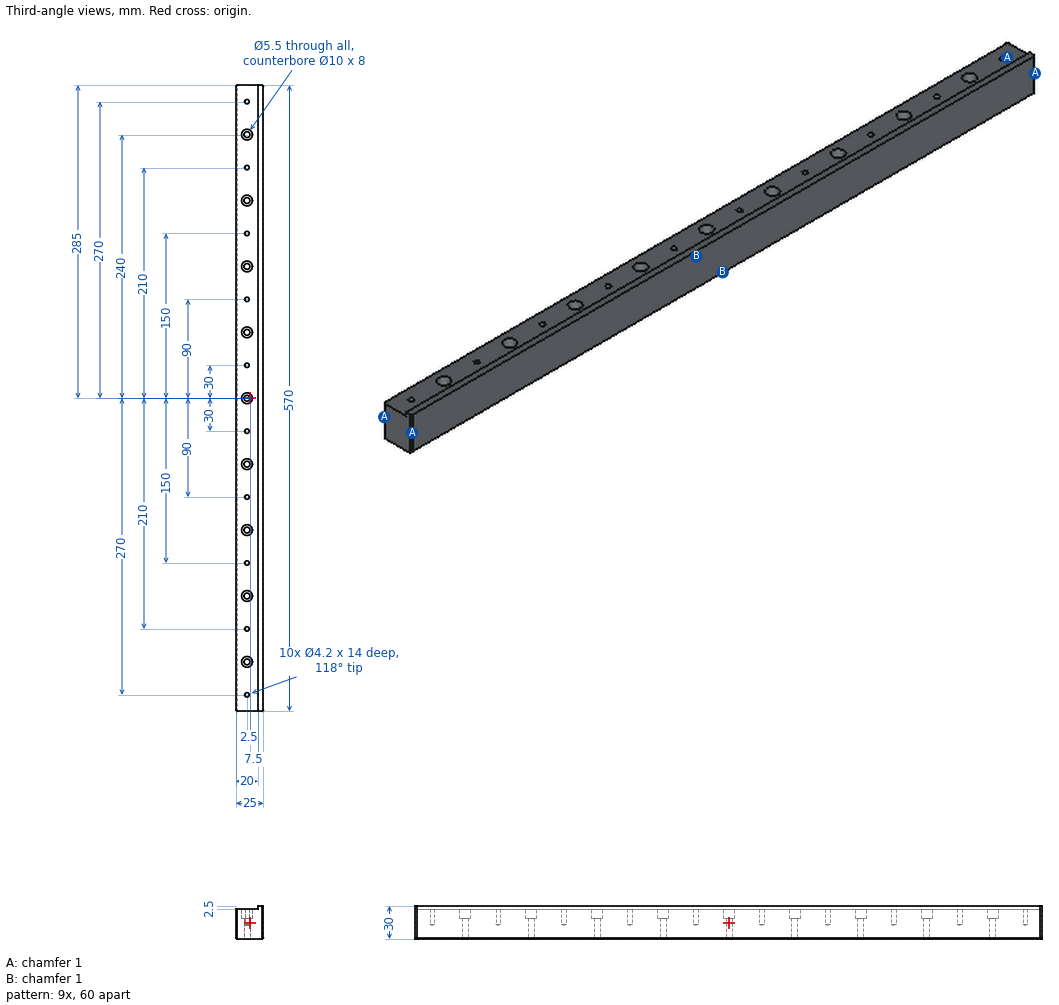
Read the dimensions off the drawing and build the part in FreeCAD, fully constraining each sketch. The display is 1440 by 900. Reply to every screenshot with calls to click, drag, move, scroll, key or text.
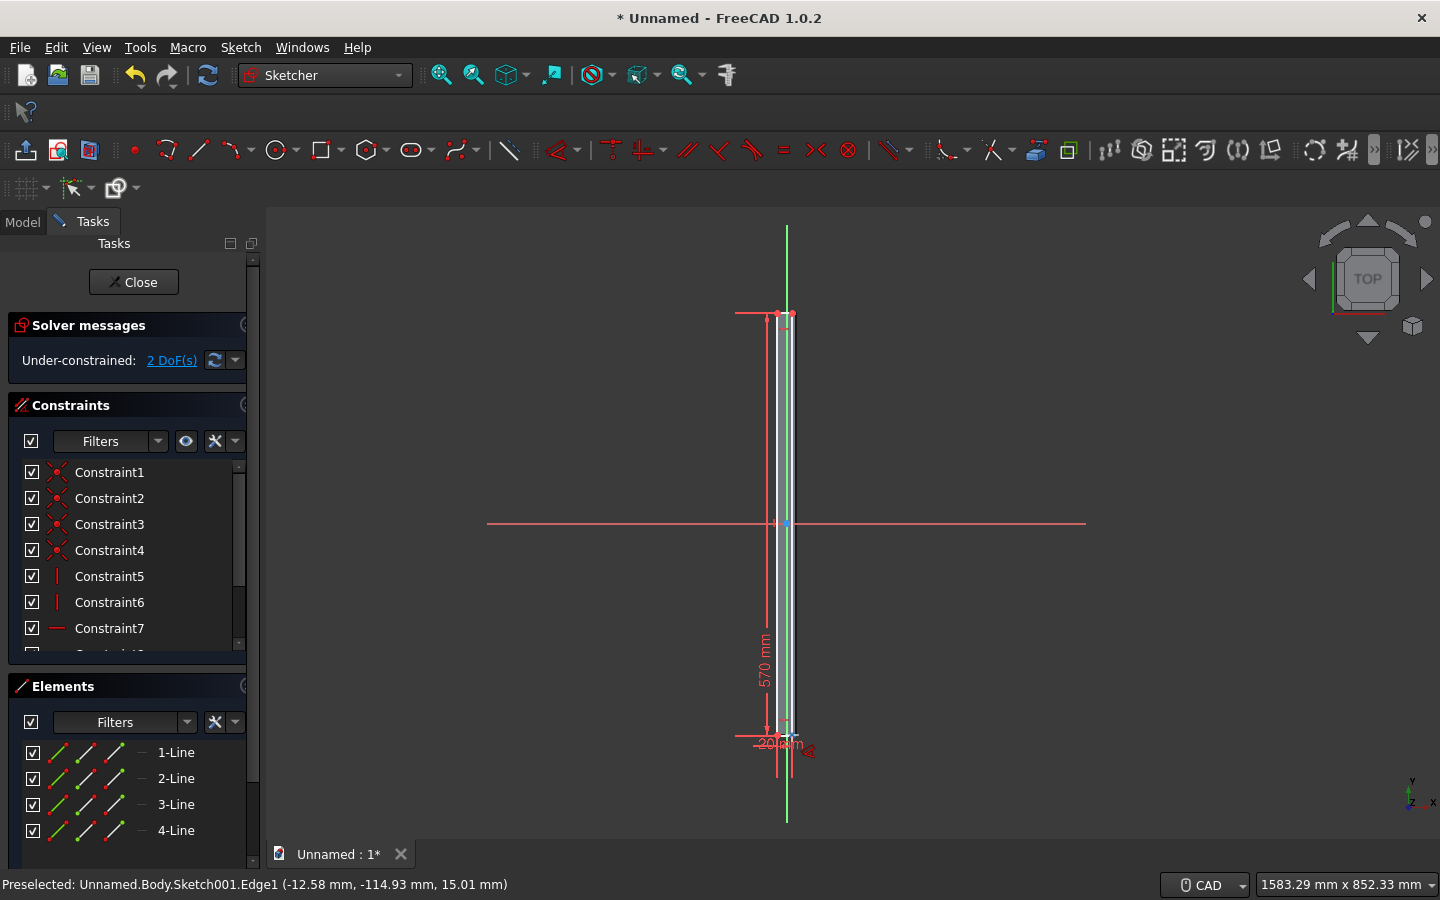
click(777, 313)
click(743, 418)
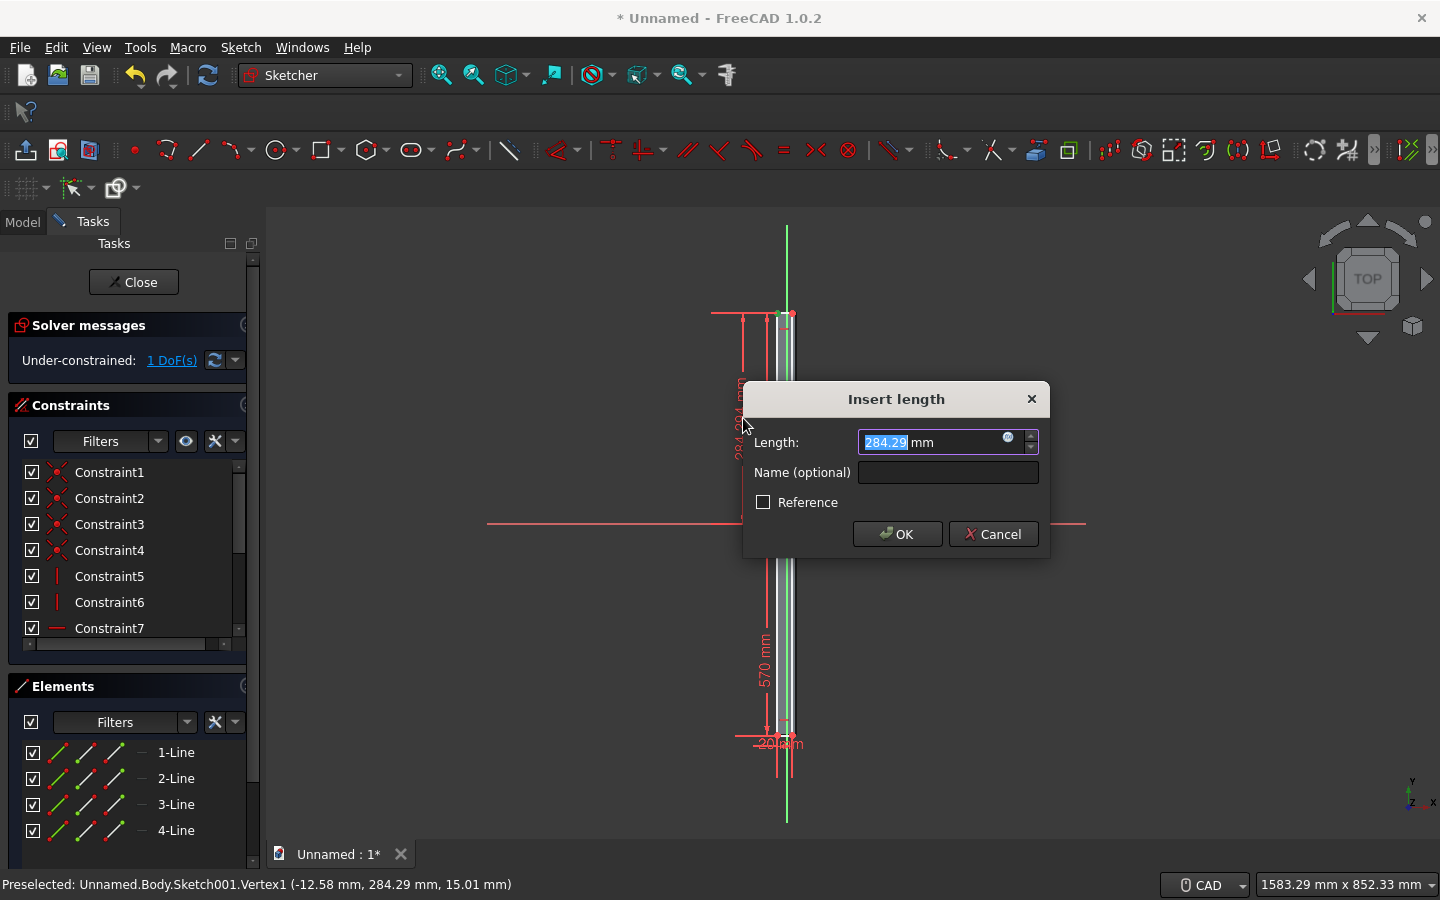
text(285)
key(Return)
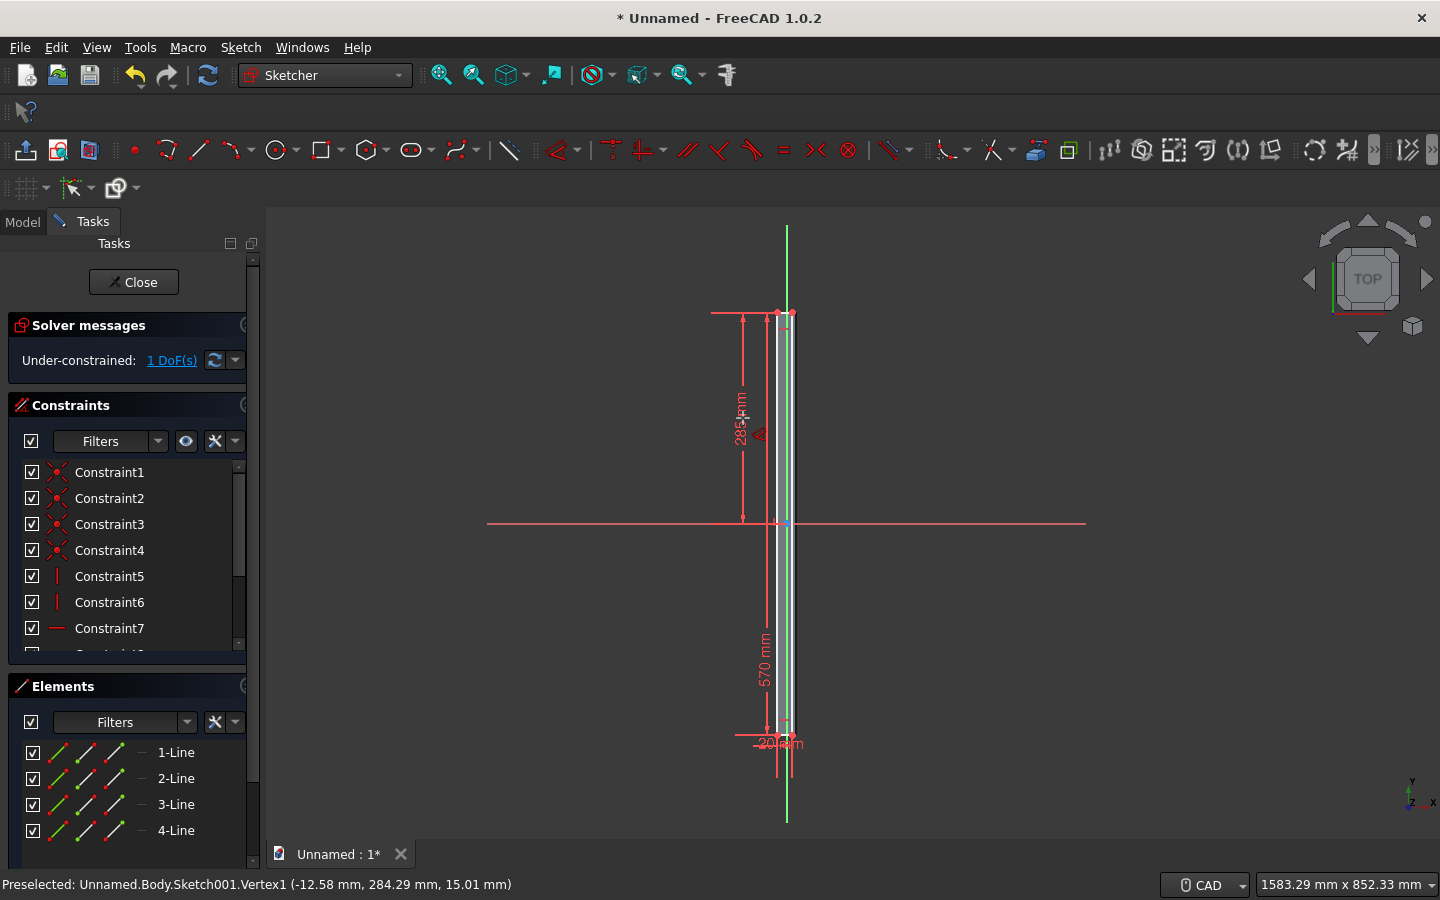
scroll(792, 735, up, 10)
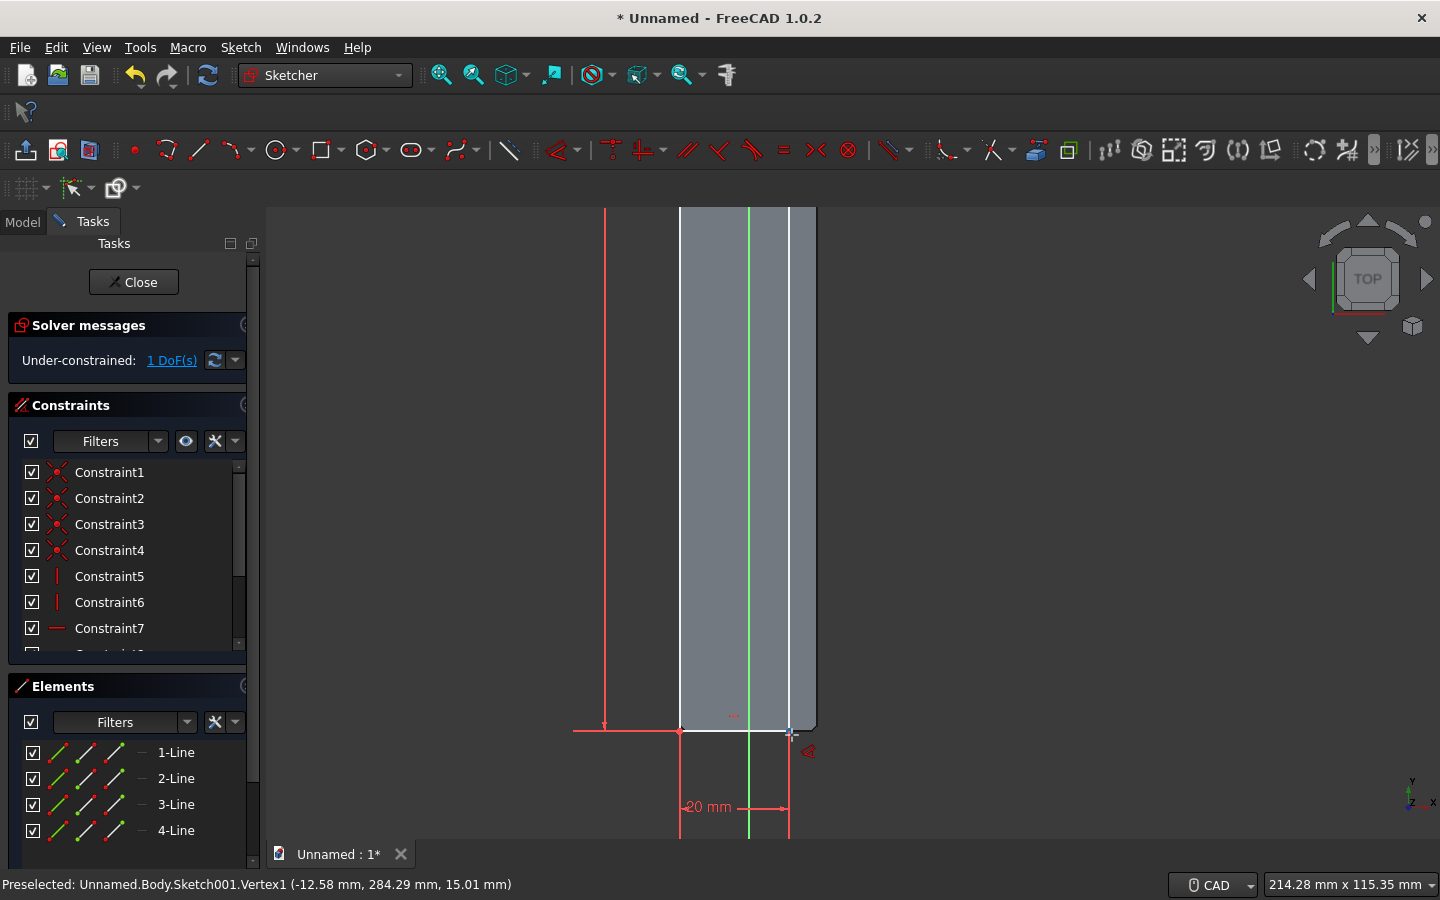
click(789, 731)
click(769, 765)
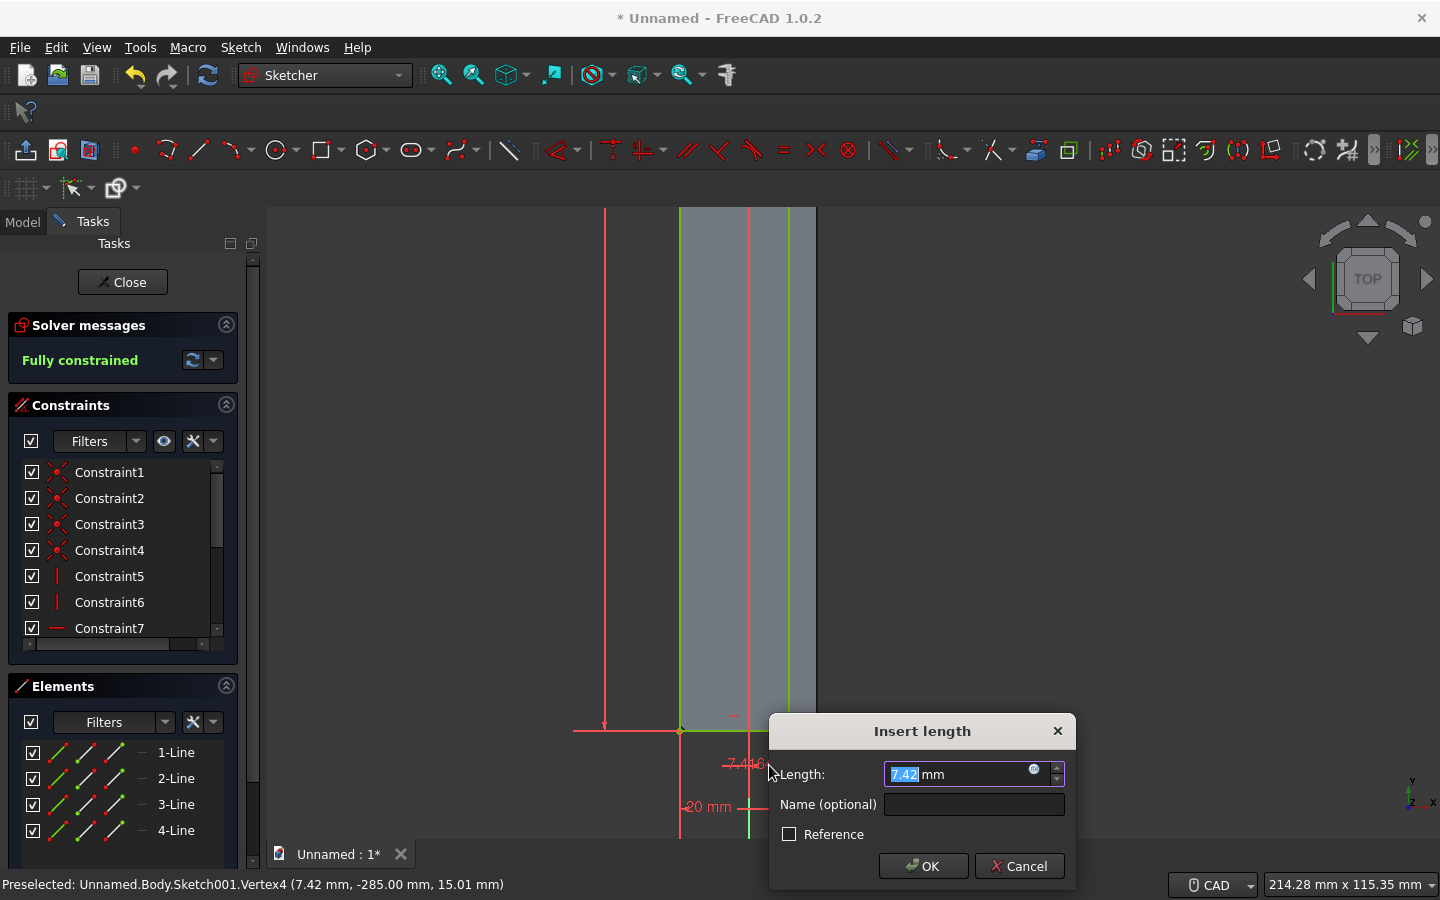
text(7.5)
key(Return)
key(Escape)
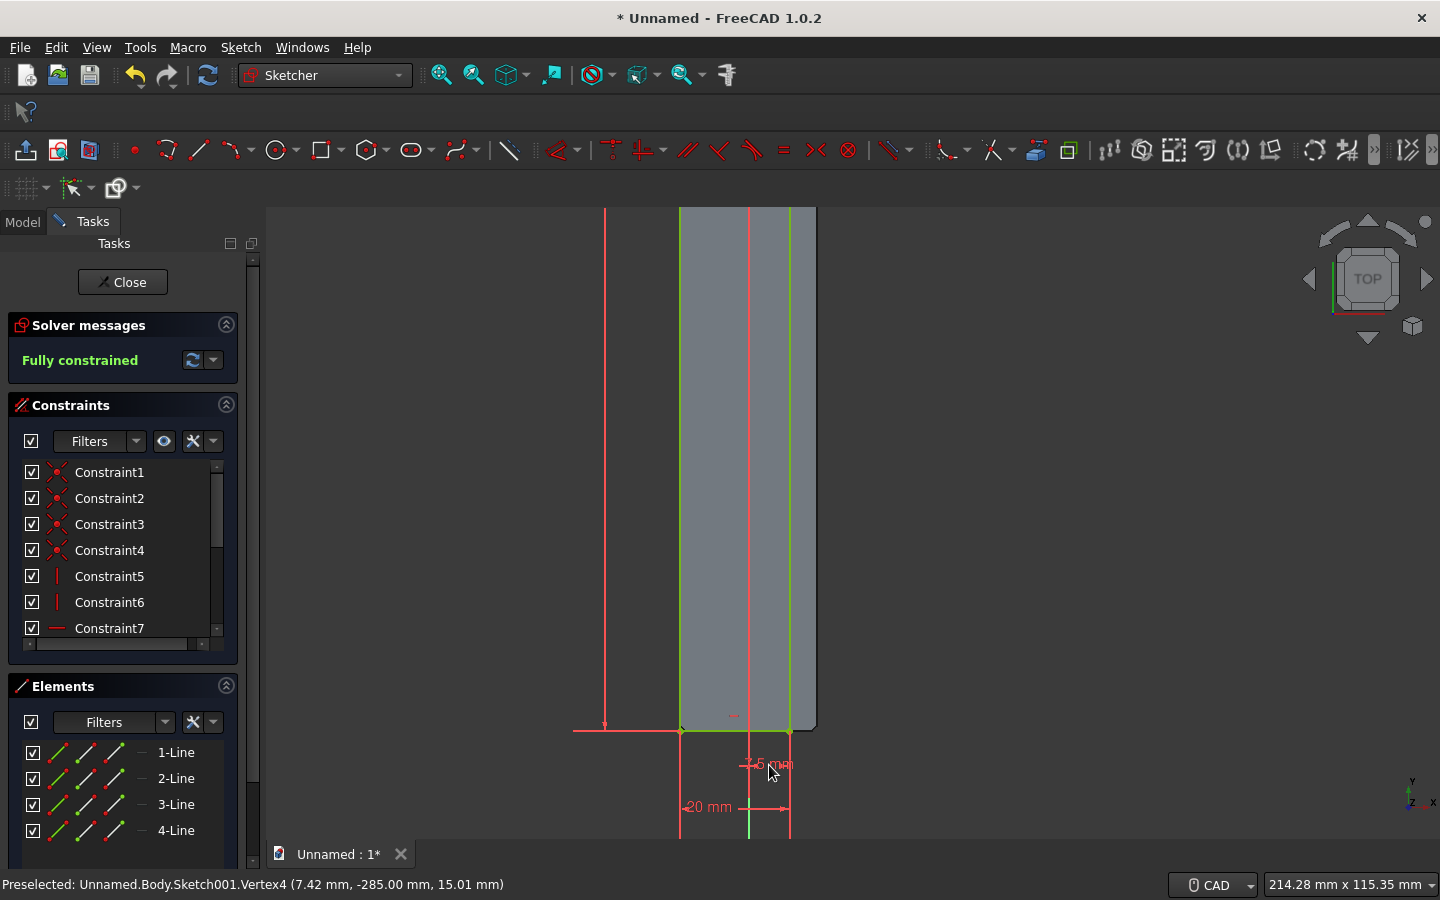
click(123, 282)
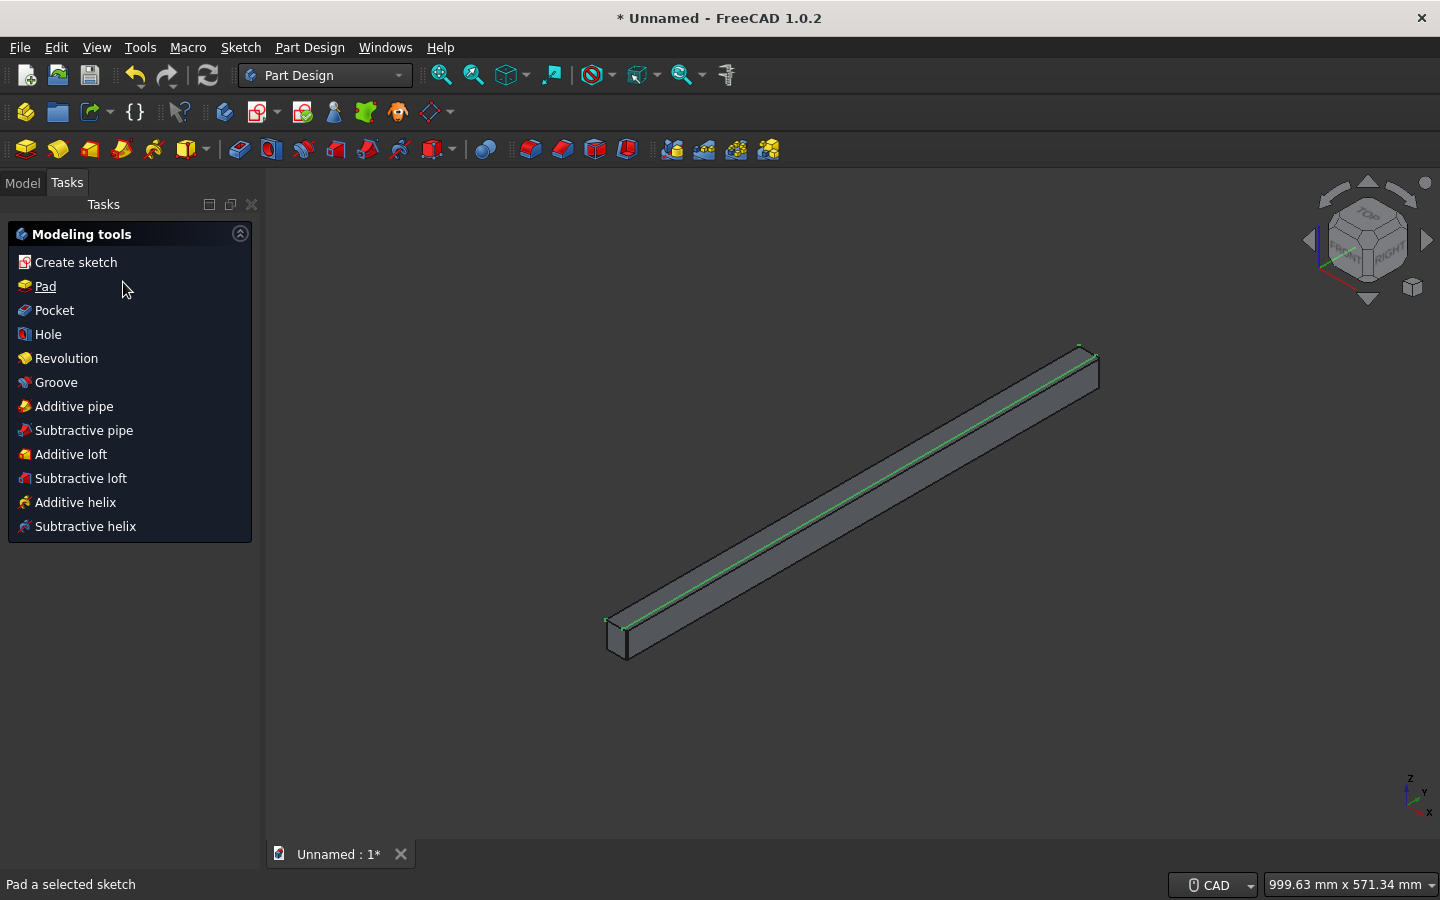
click(240, 150)